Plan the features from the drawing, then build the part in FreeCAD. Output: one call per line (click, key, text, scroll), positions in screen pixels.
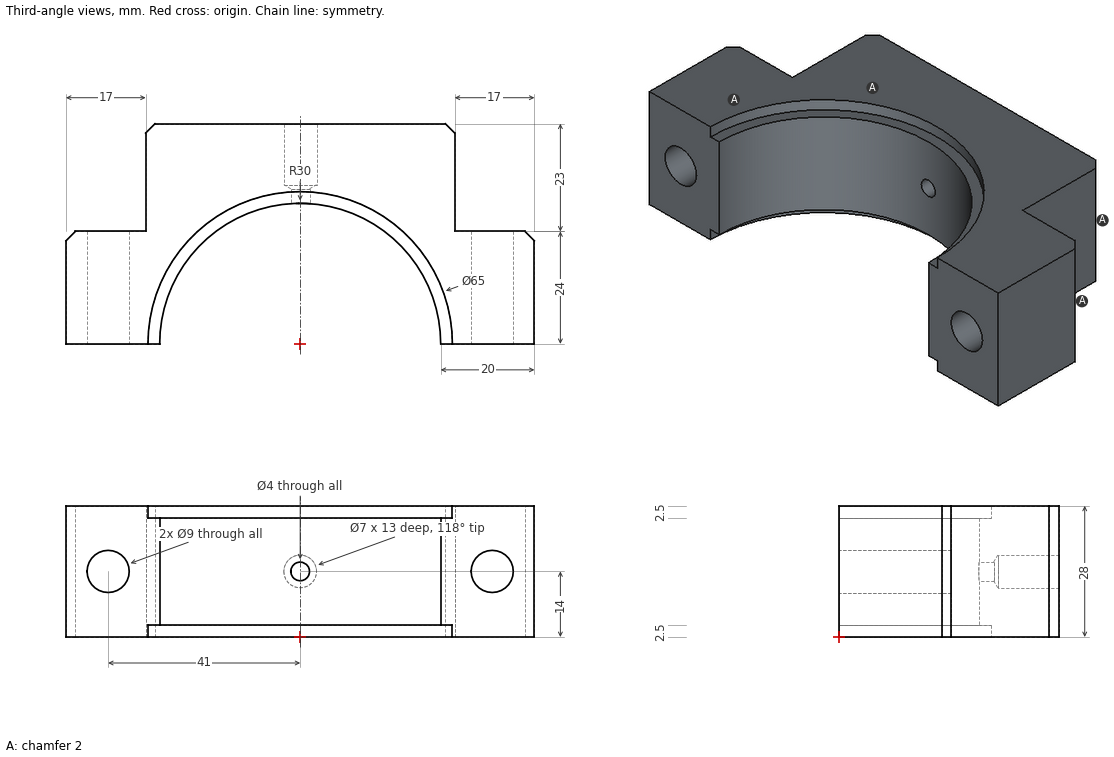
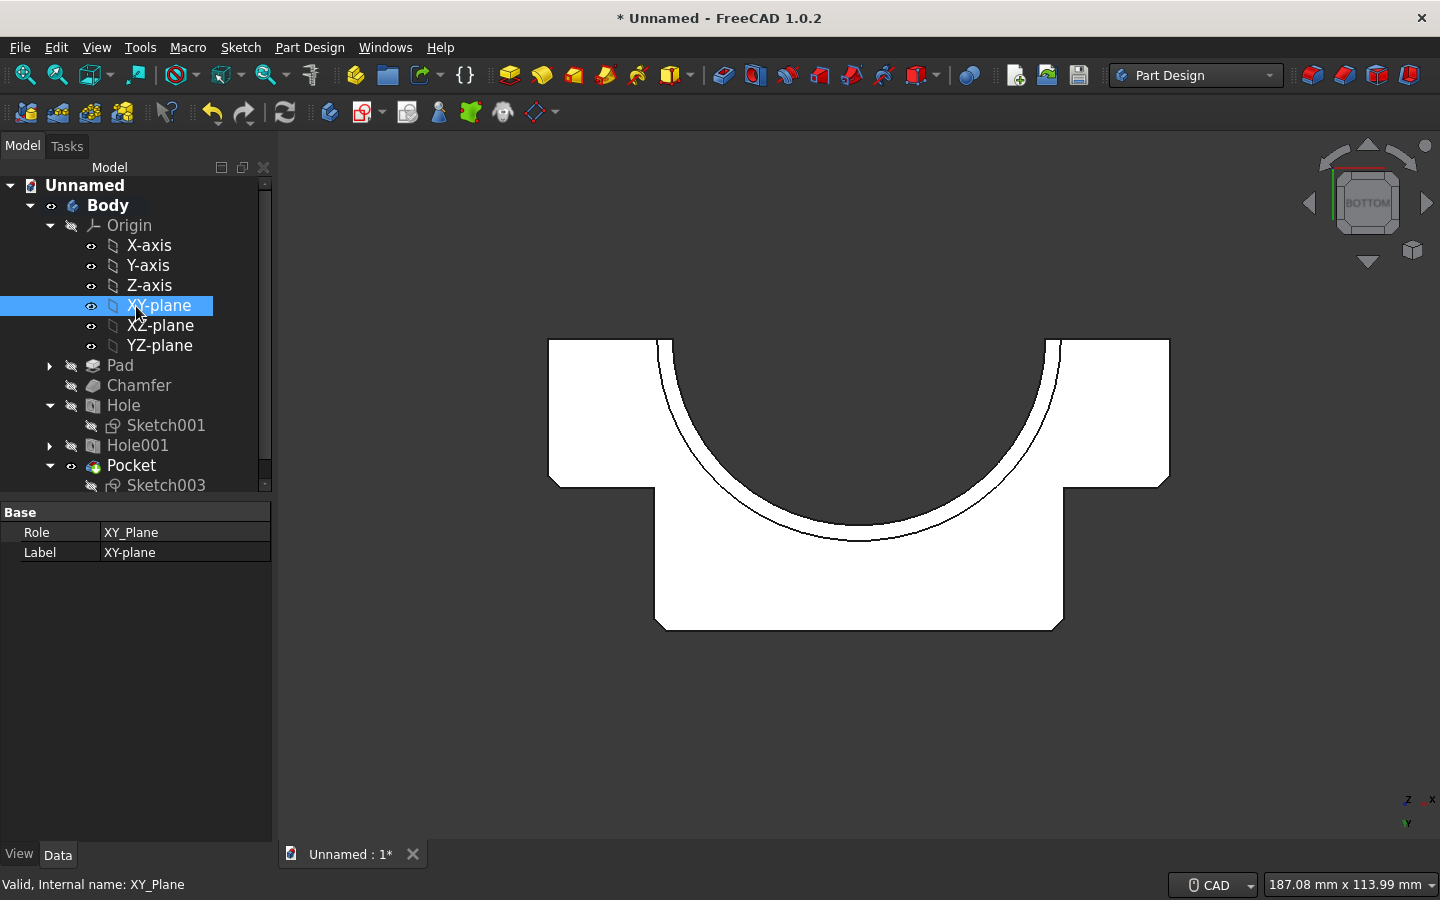
click(536, 112)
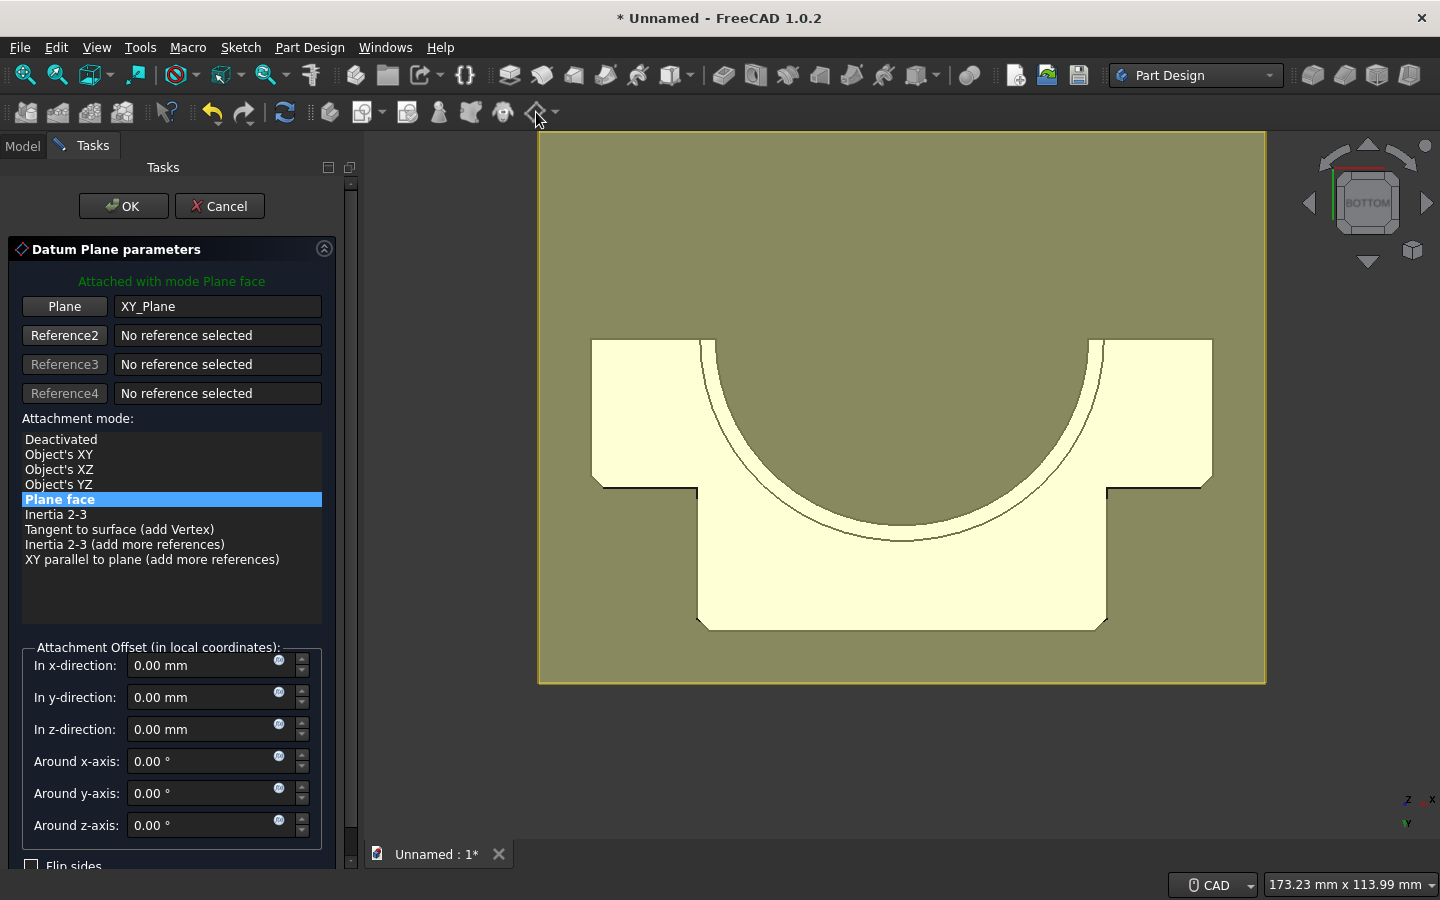
triple_click(210, 729)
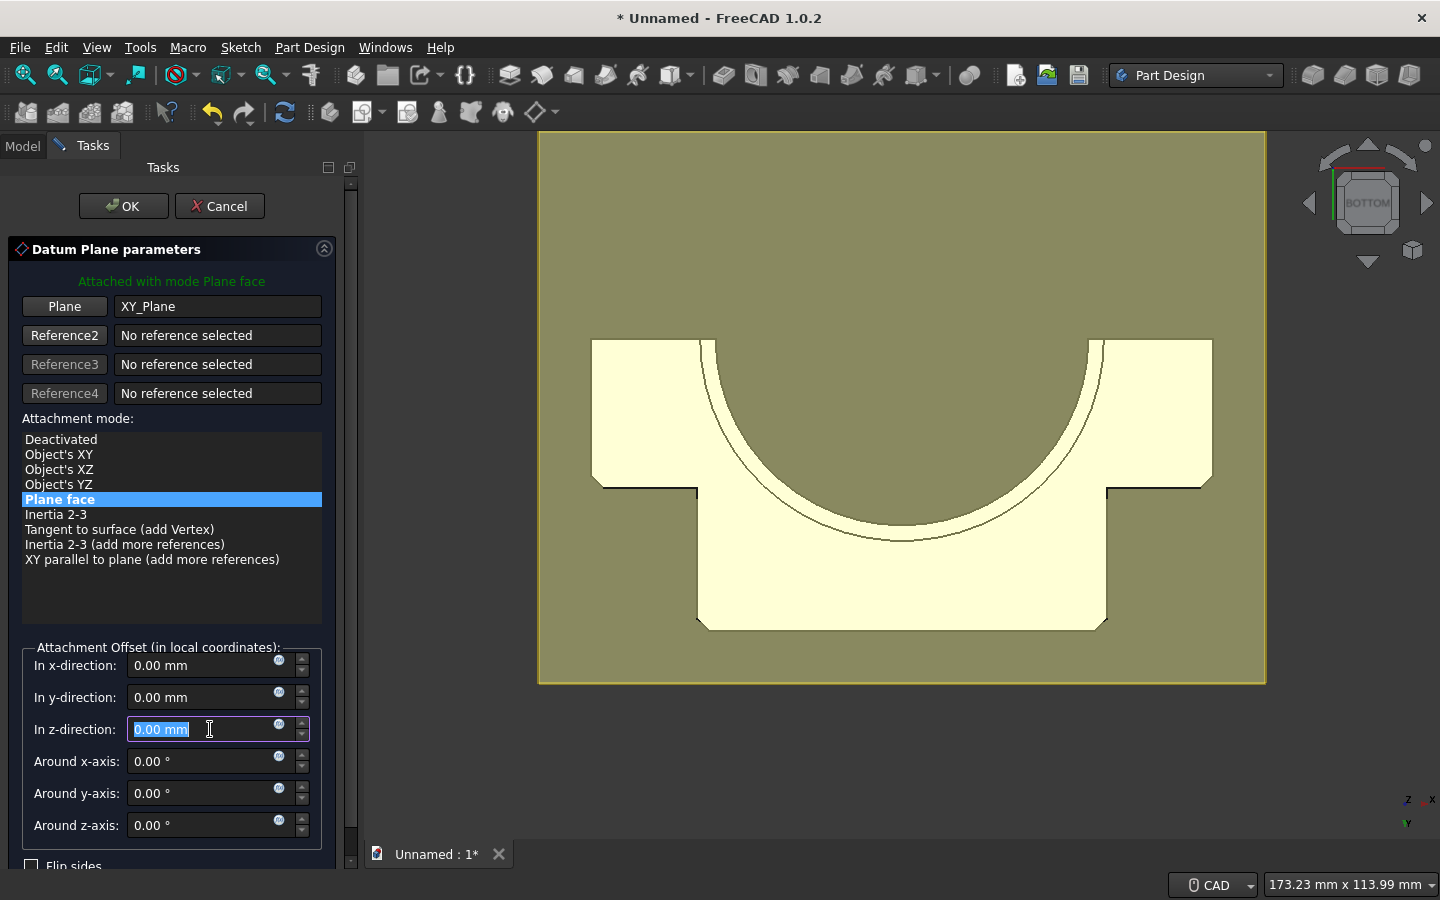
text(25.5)
key(Tab)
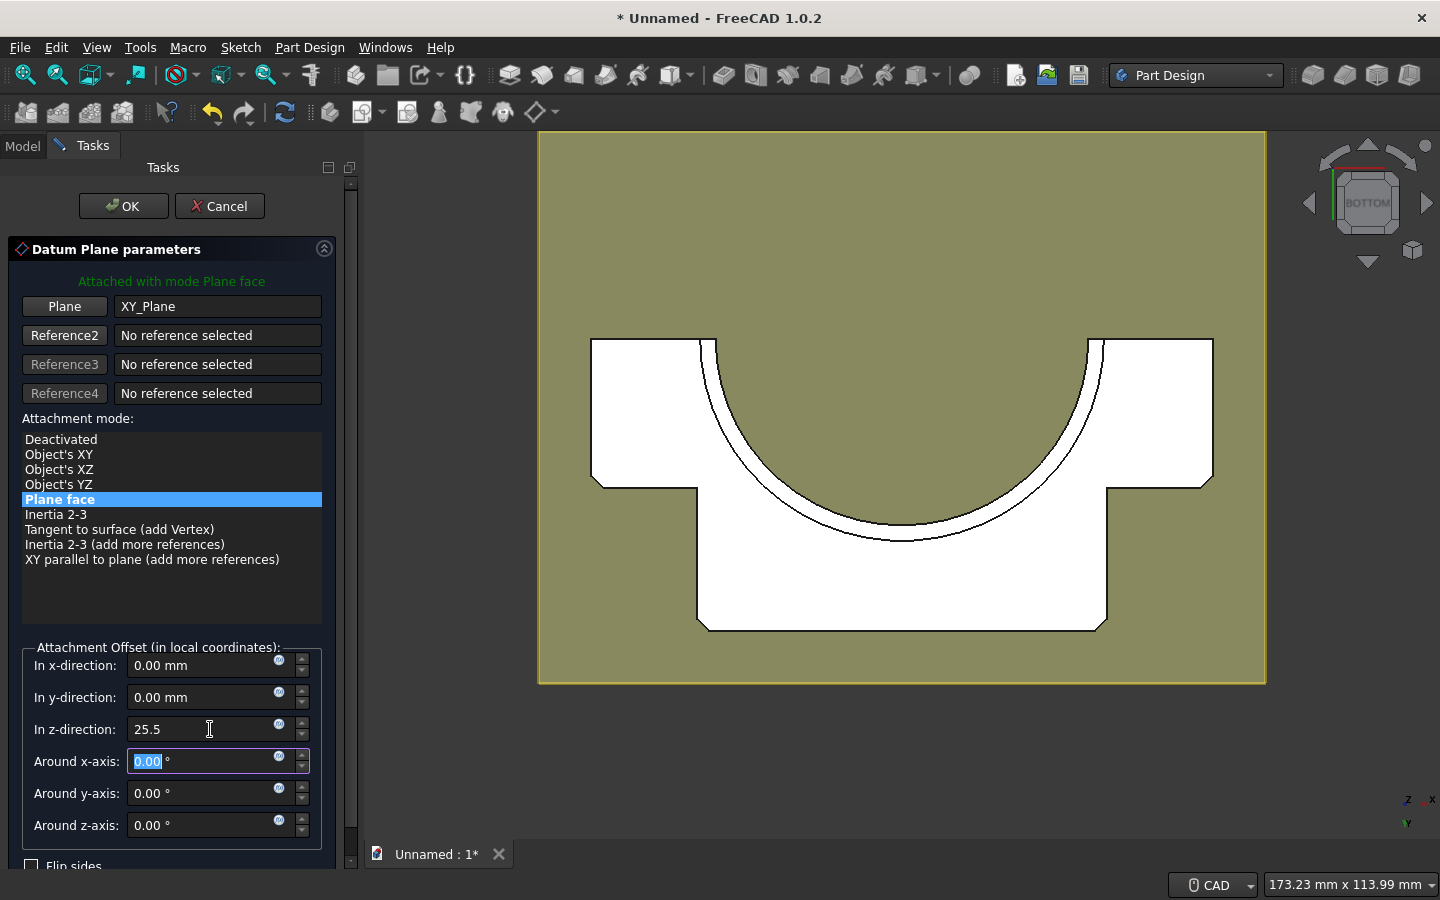
click(124, 206)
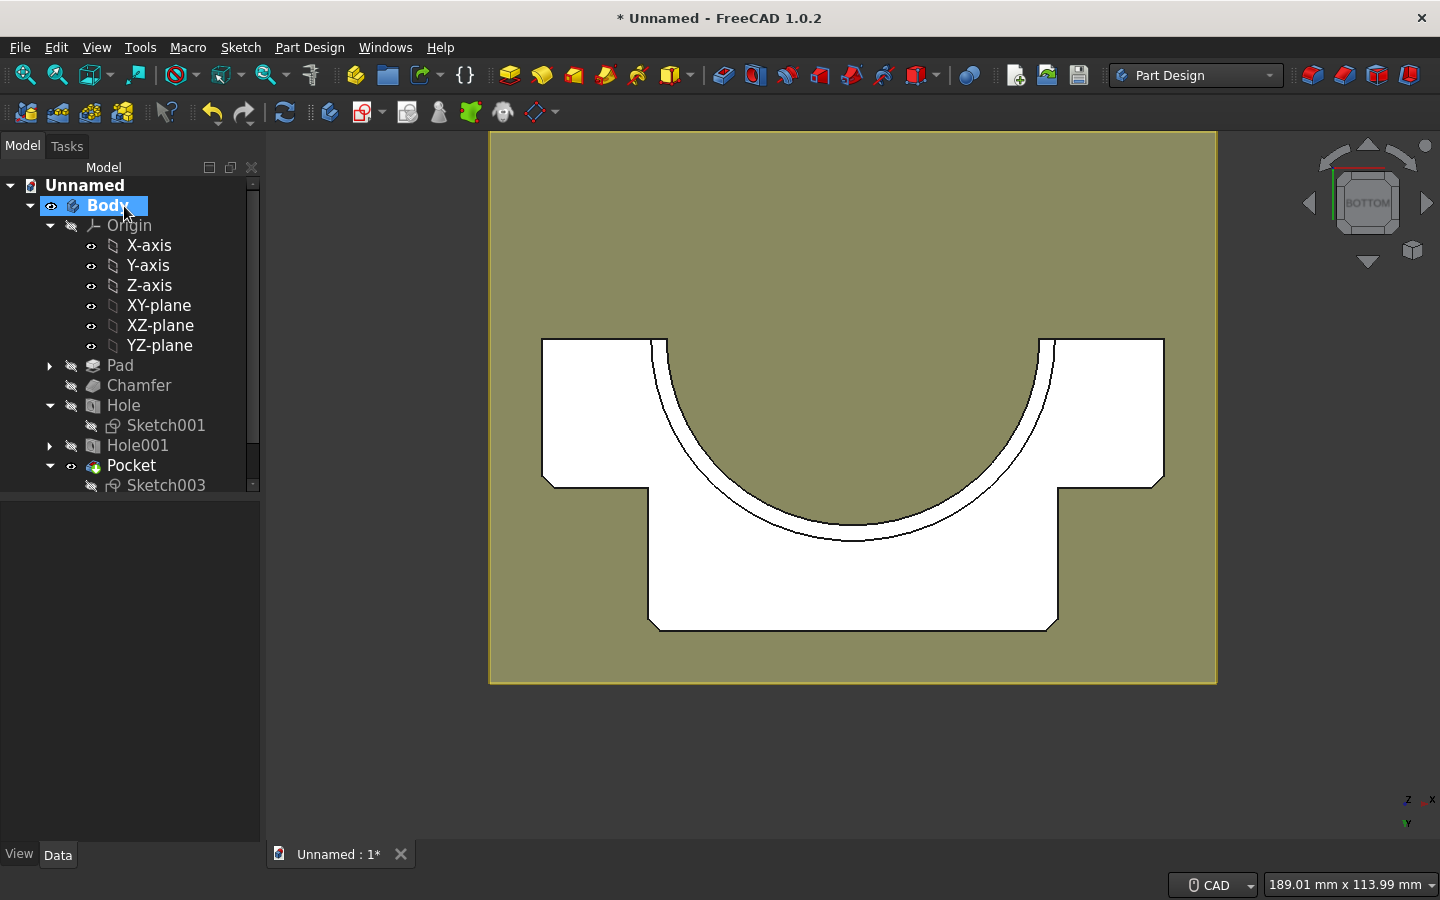
scroll(100, 341, down, 3)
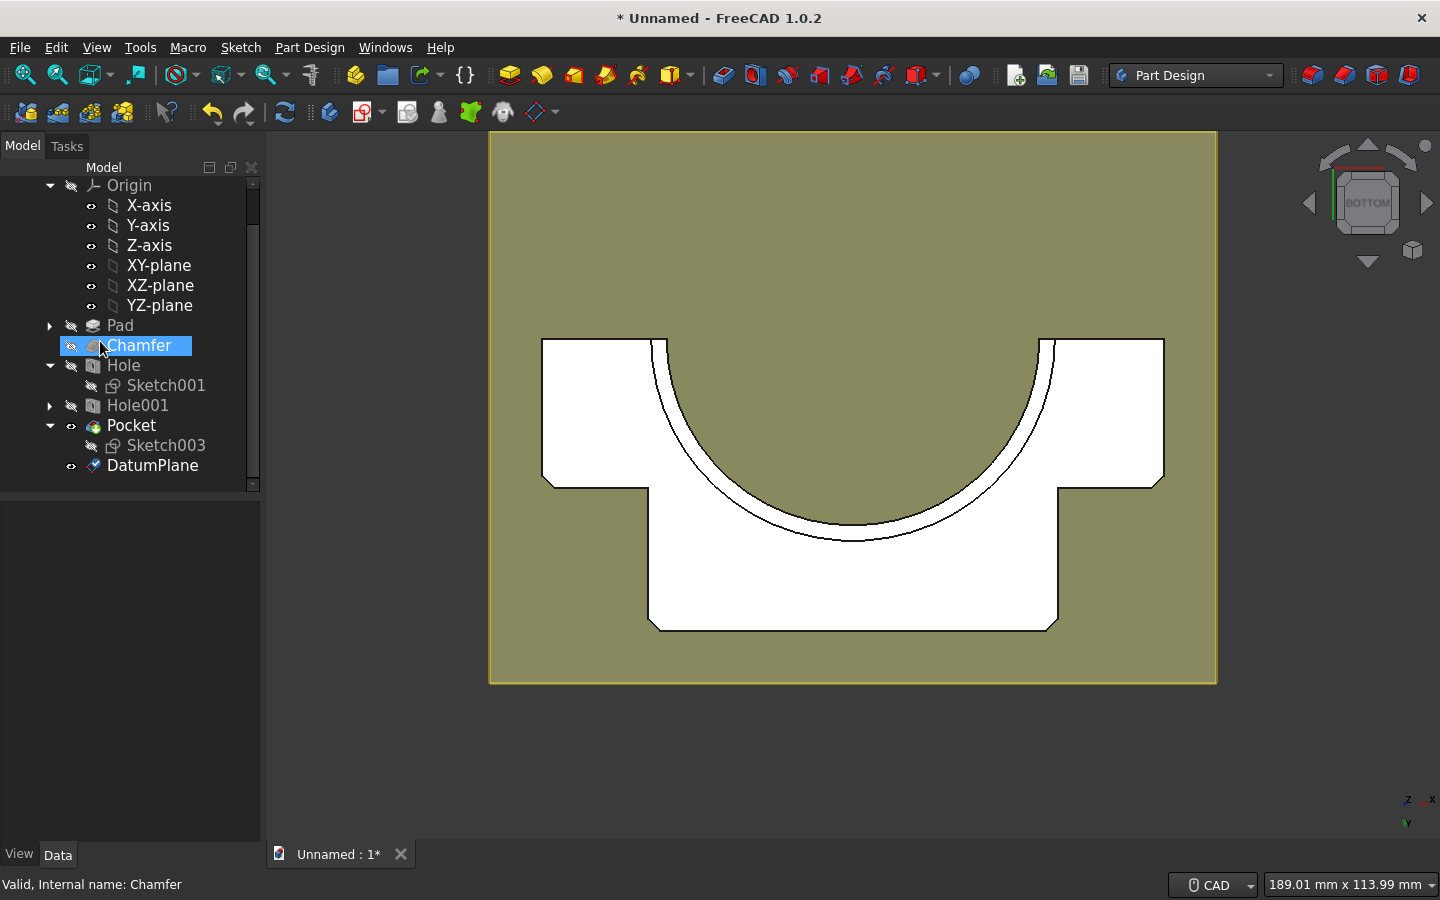
click(116, 466)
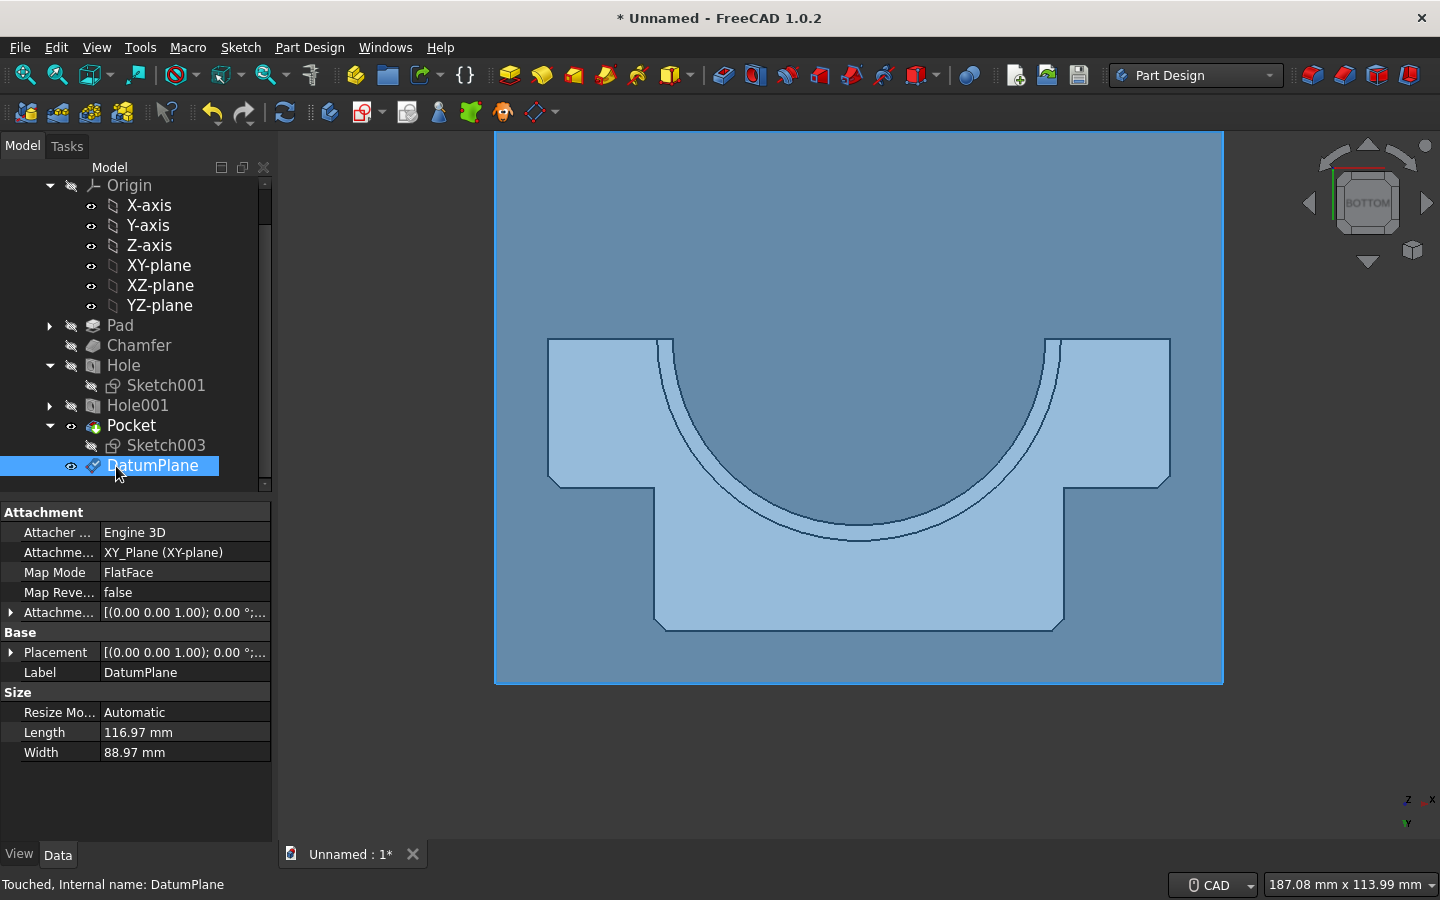
click(362, 112)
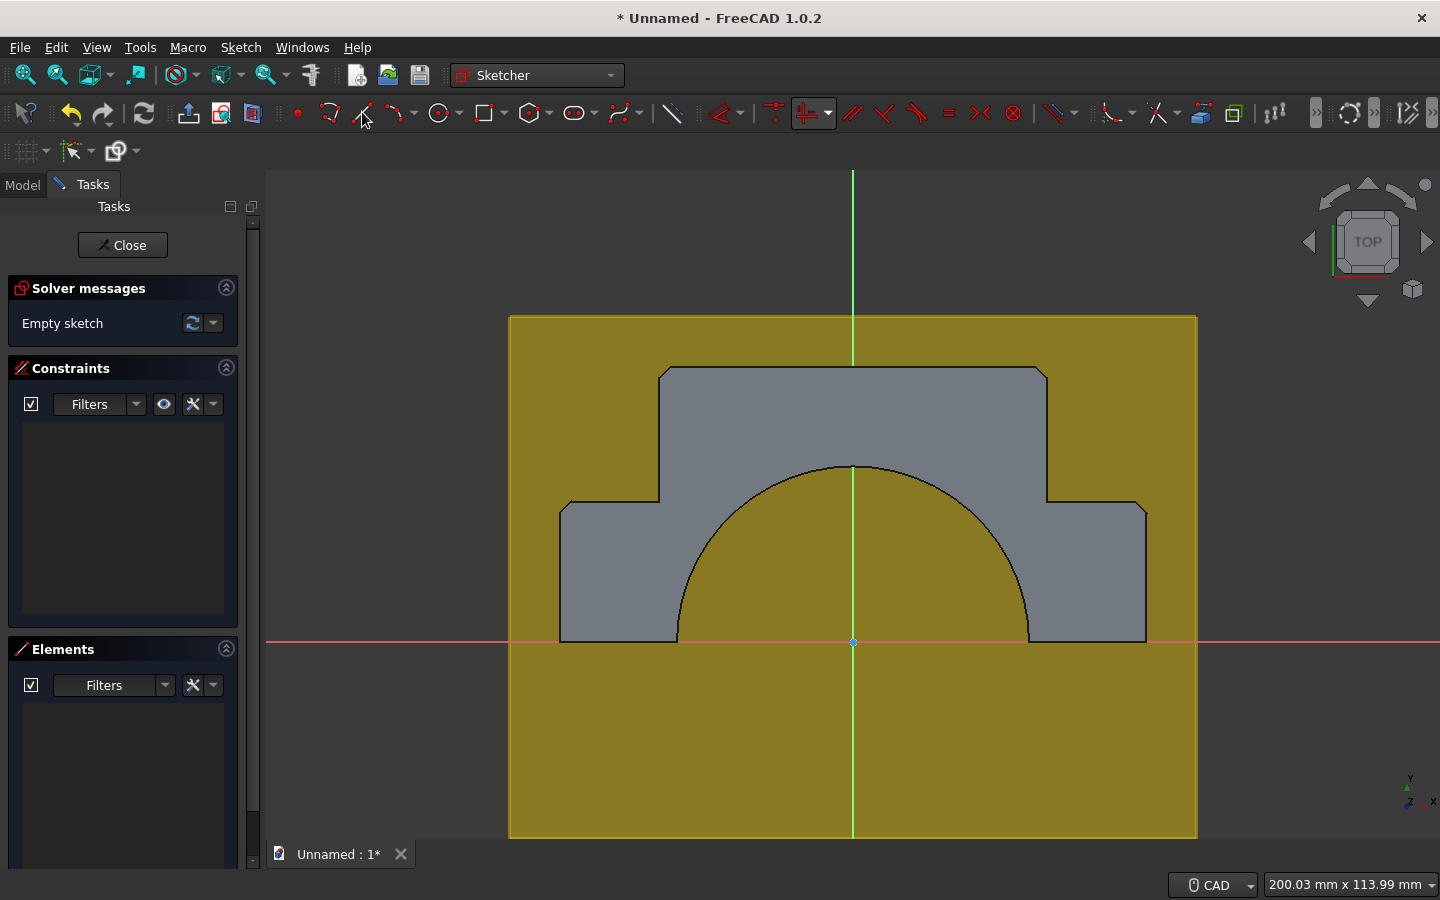
click(254, 114)